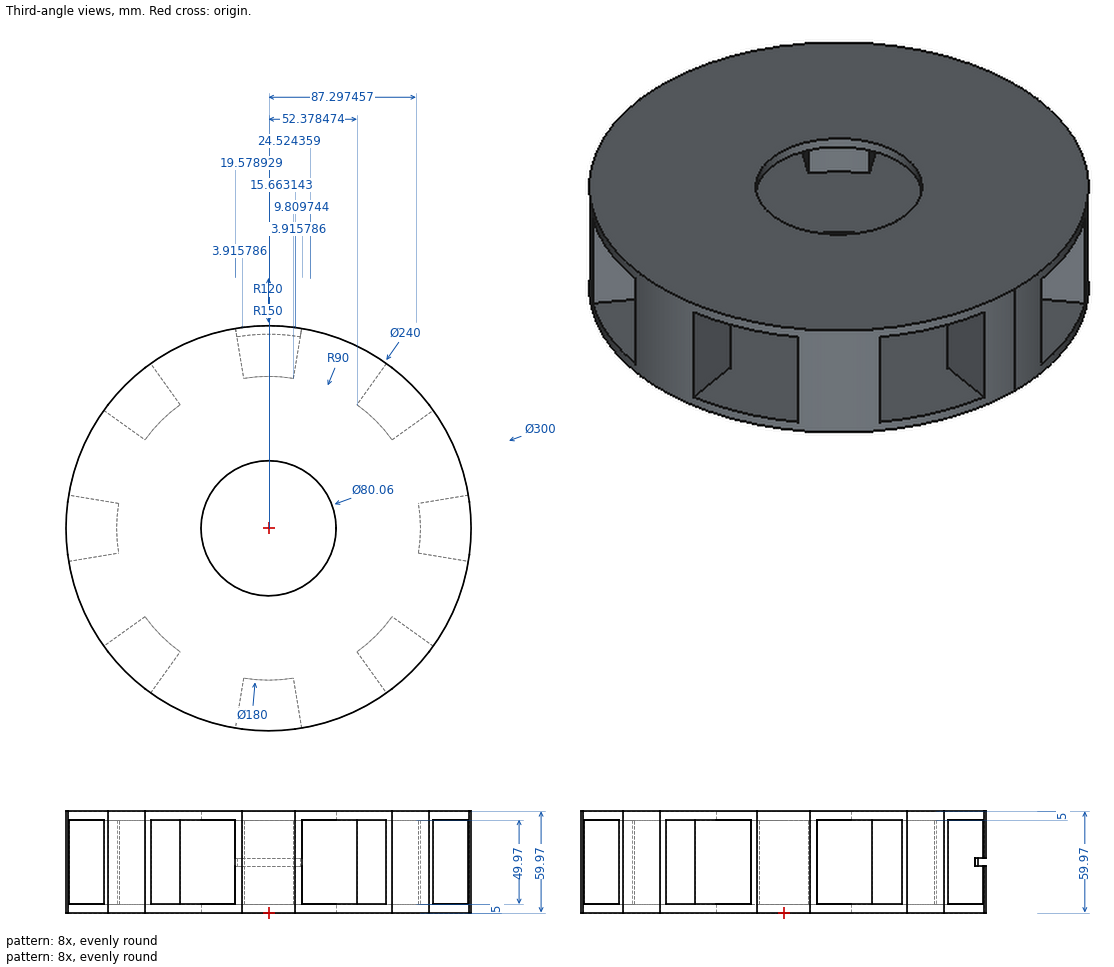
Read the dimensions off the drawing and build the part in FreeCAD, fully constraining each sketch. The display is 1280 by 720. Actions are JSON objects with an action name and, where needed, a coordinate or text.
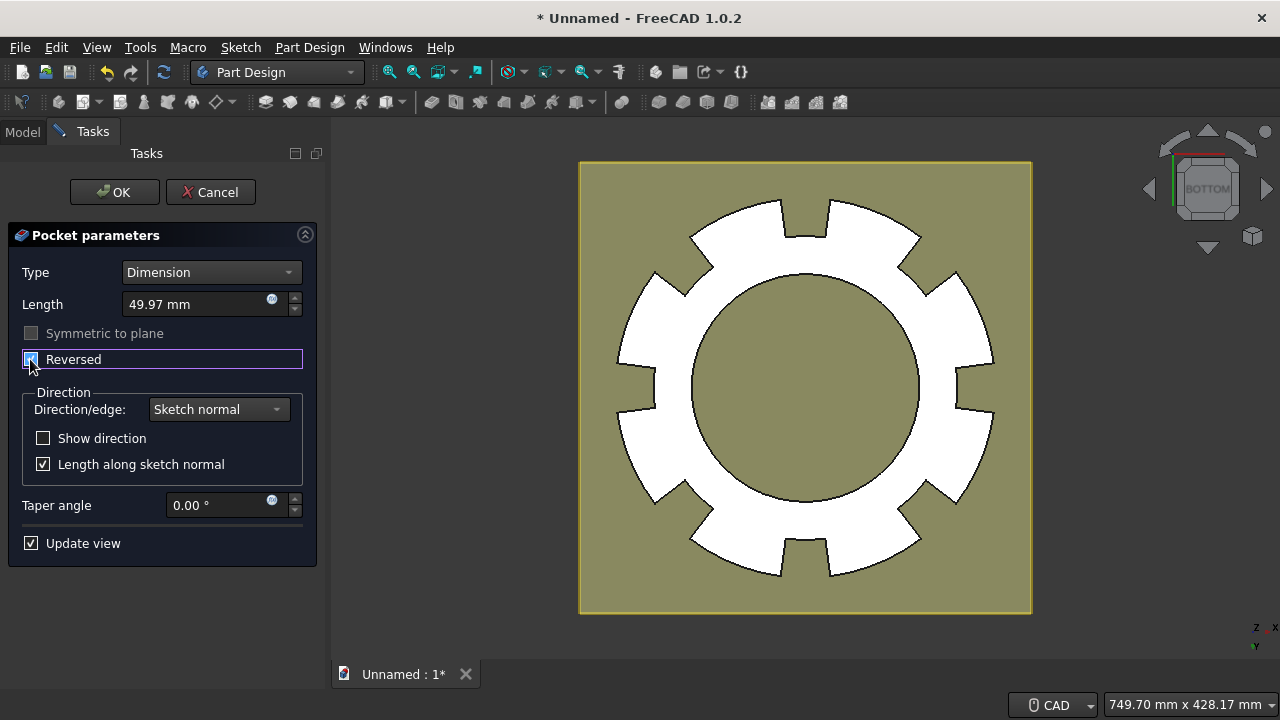
{"action": "left_click", "coordinate": [115, 192]}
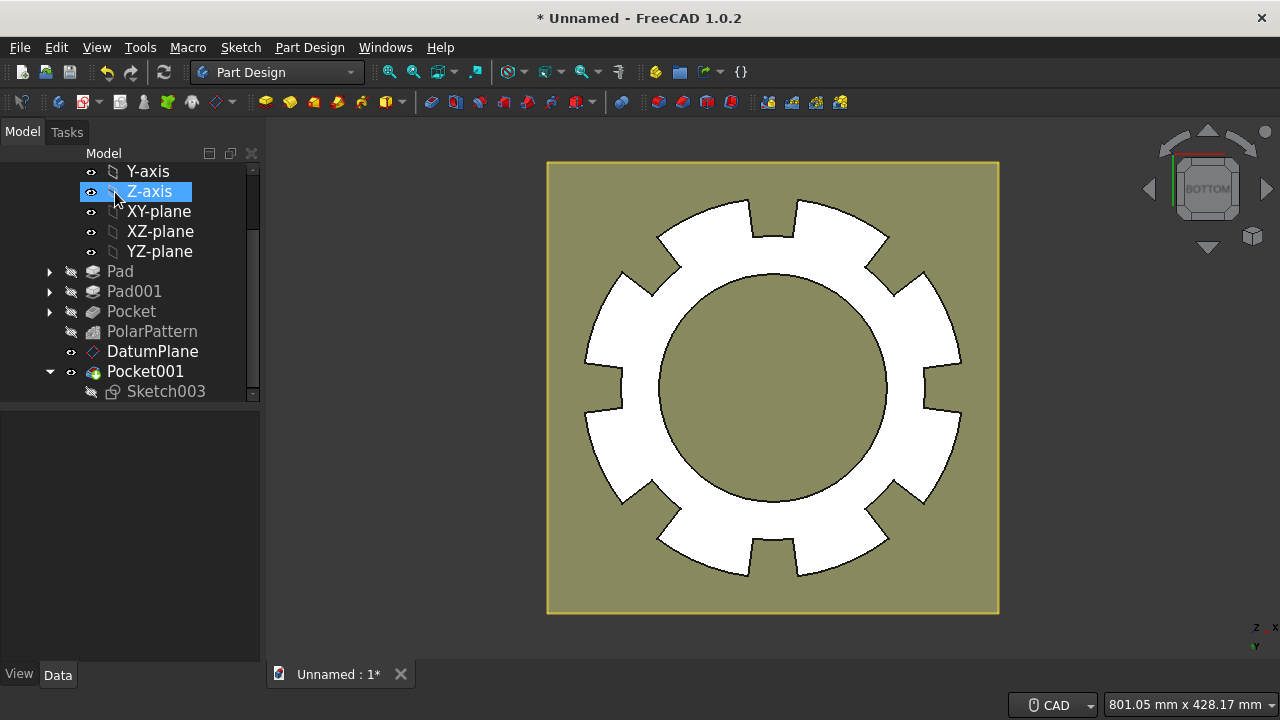
{"action": "left_click", "coordinate": [116, 352]}
{"action": "key", "text": "space"}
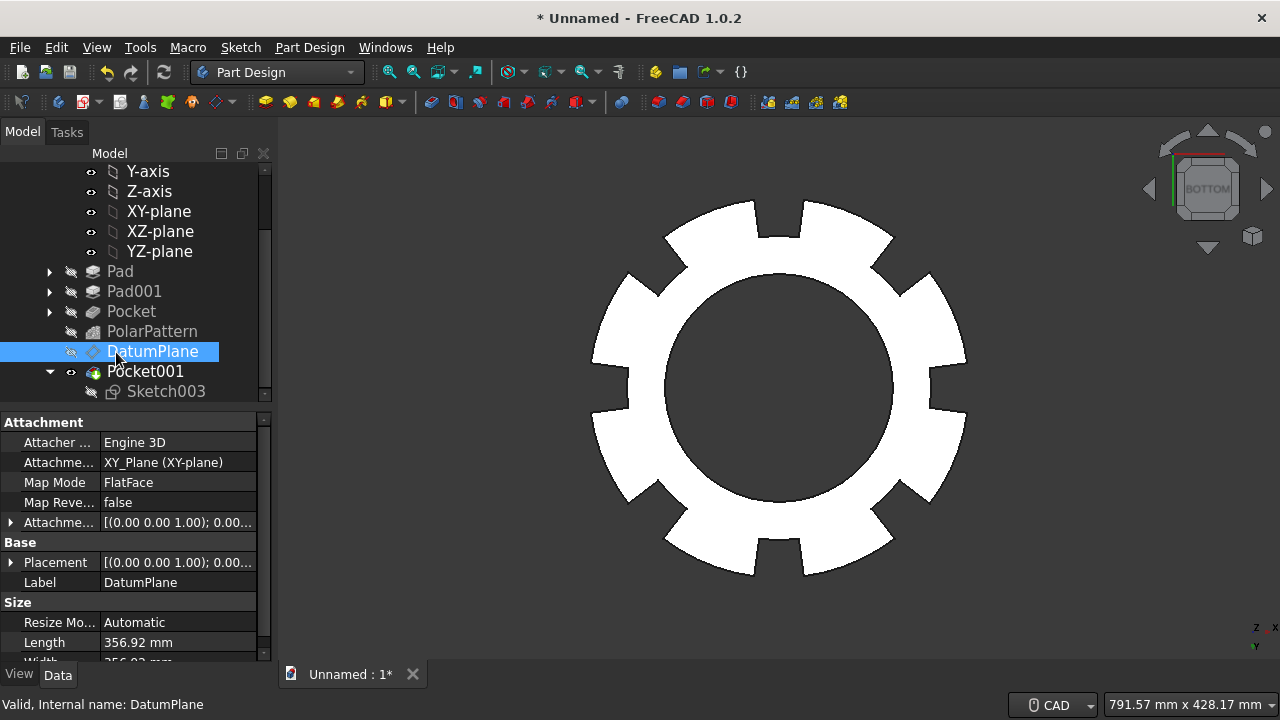
{"action": "left_click", "coordinate": [116, 372]}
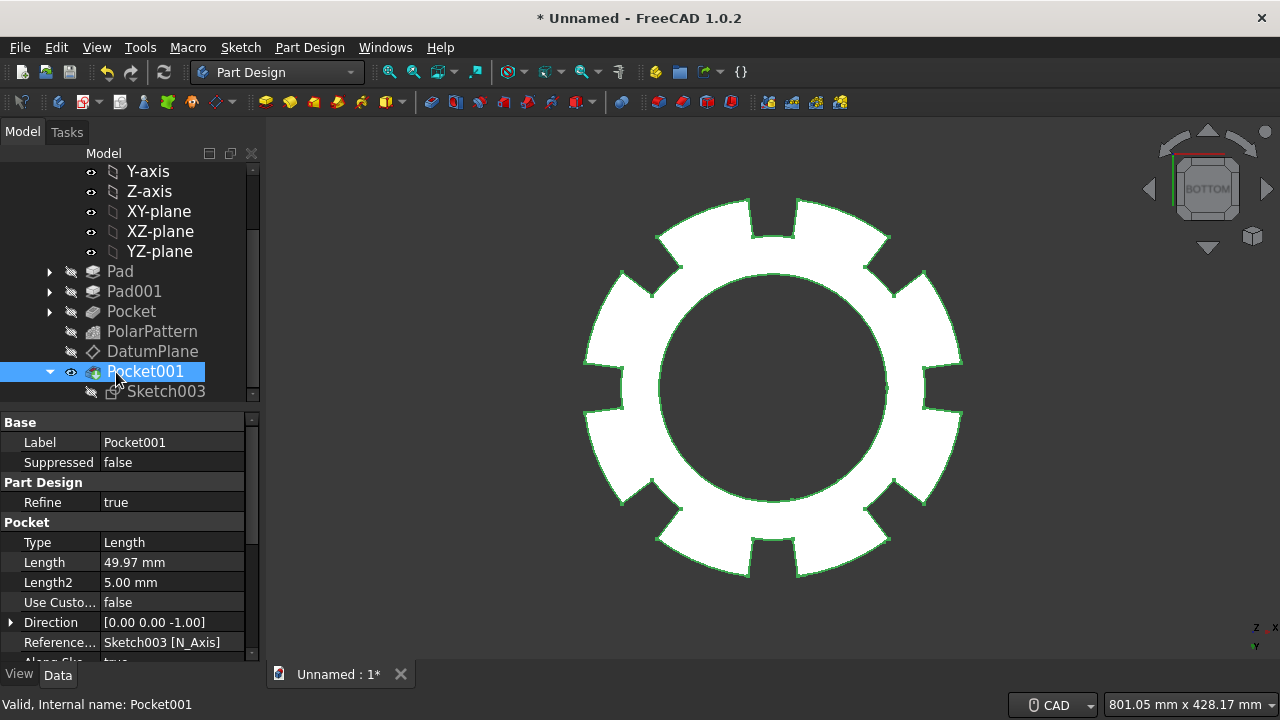
{"action": "left_click", "coordinate": [816, 102]}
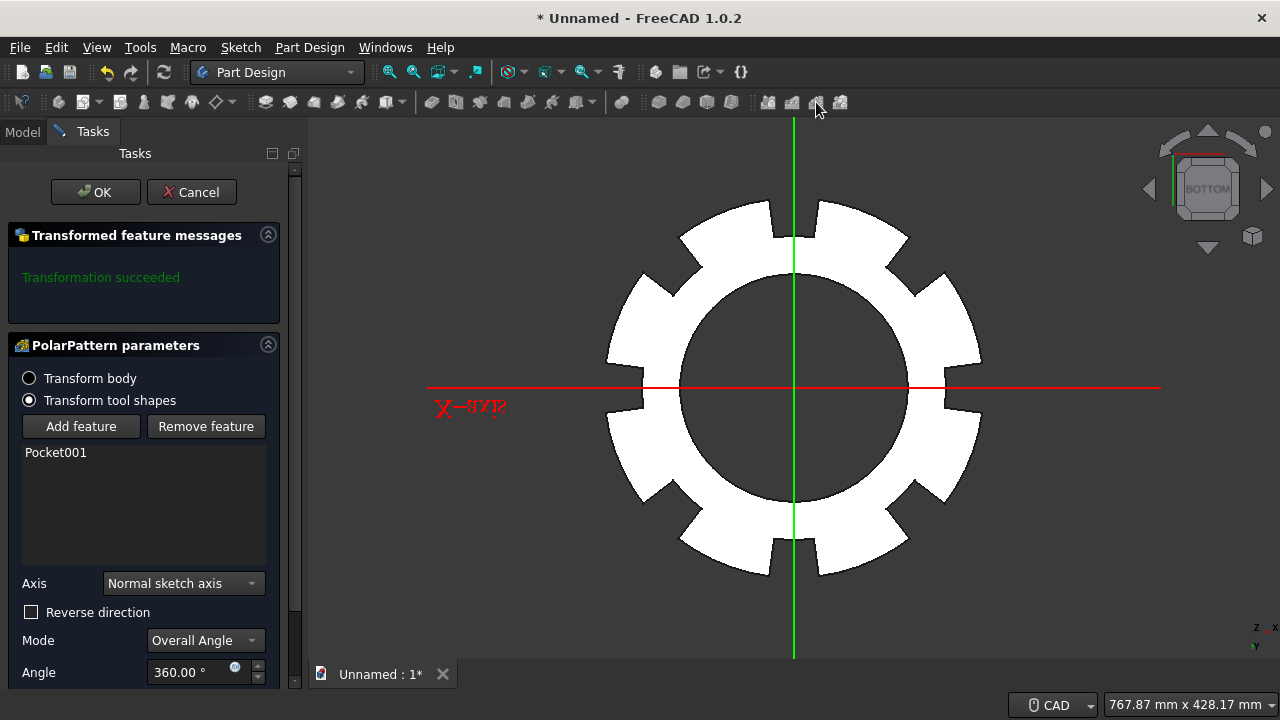
{"action": "left_click", "coordinate": [184, 584]}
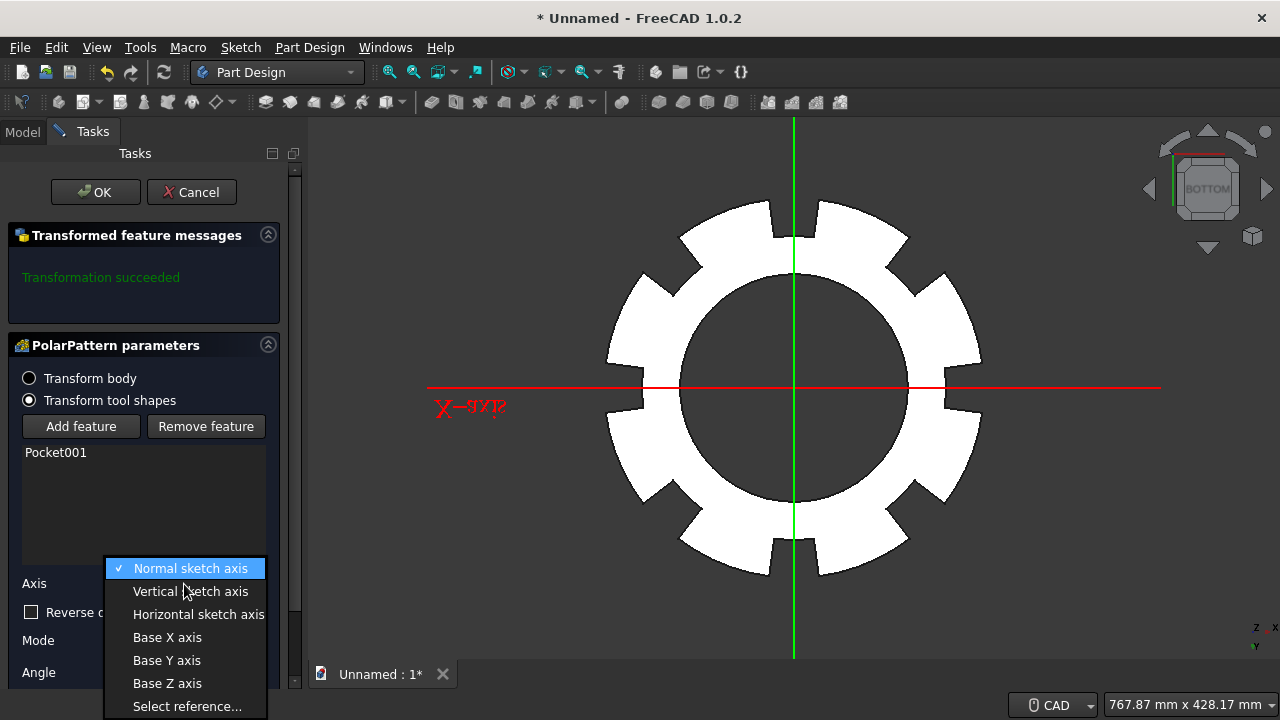
{"action": "left_click", "coordinate": [184, 684]}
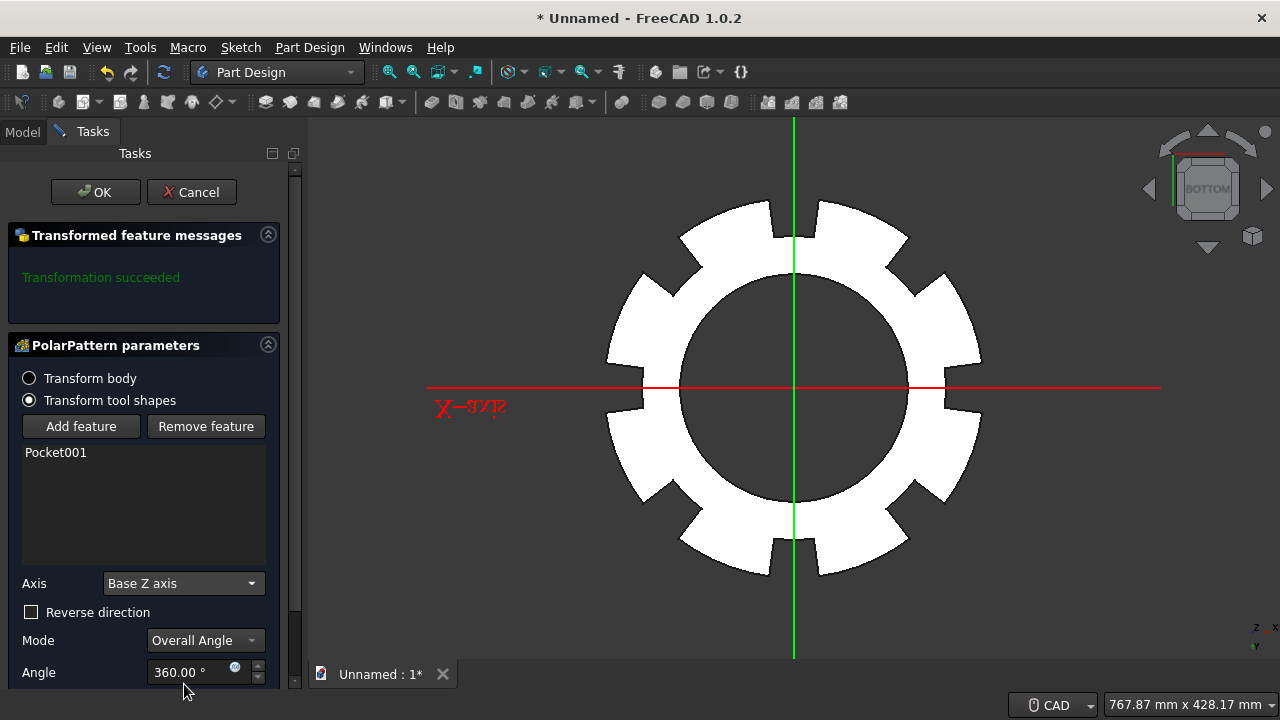
{"action": "scroll", "coordinate": [295, 426], "scroll_direction": "down", "scroll_amount": 2}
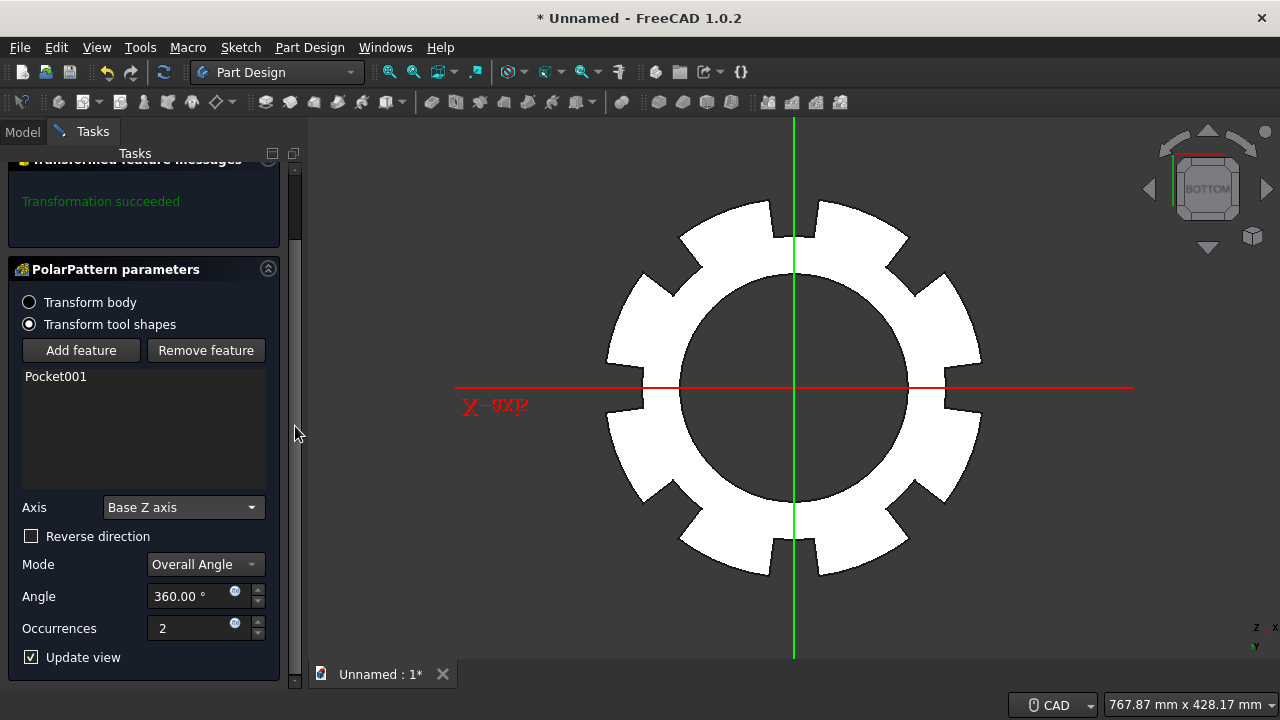
{"action": "triple_click", "coordinate": [198, 628]}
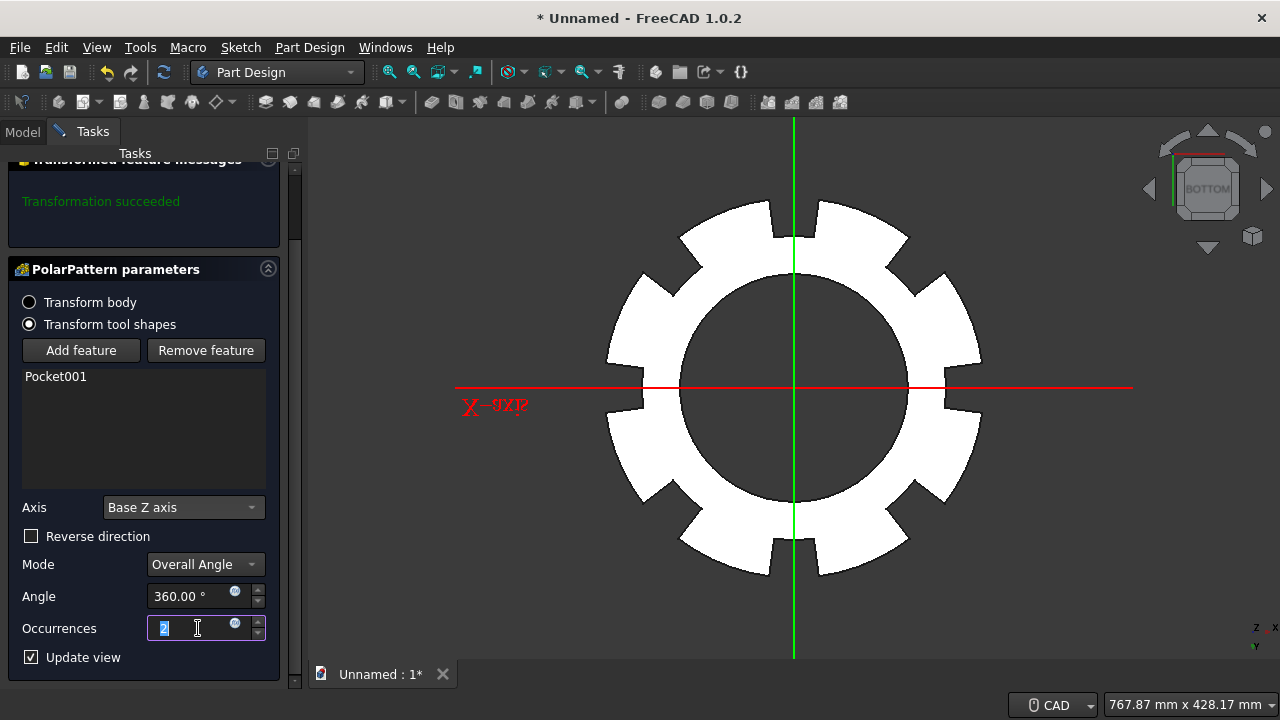
{"action": "type", "text": "8"}
{"action": "key", "text": "Tab"}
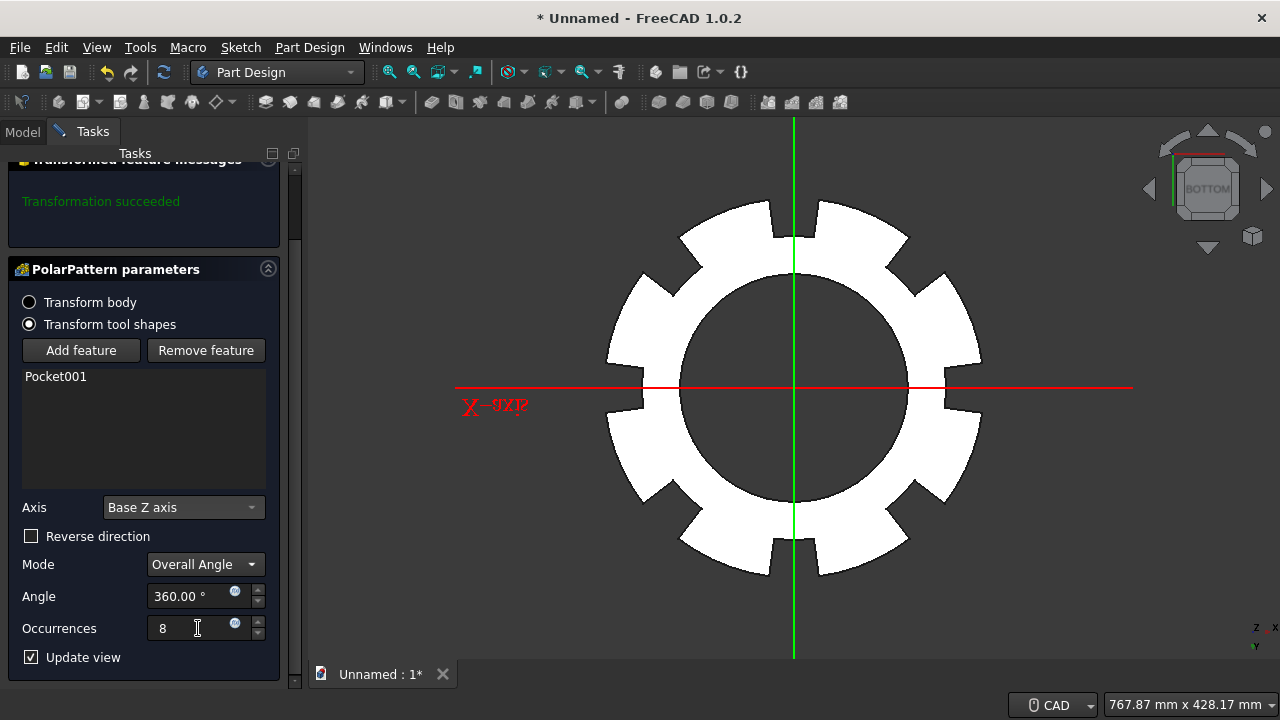
{"action": "scroll", "coordinate": [295, 426], "scroll_direction": "up", "scroll_amount": 3}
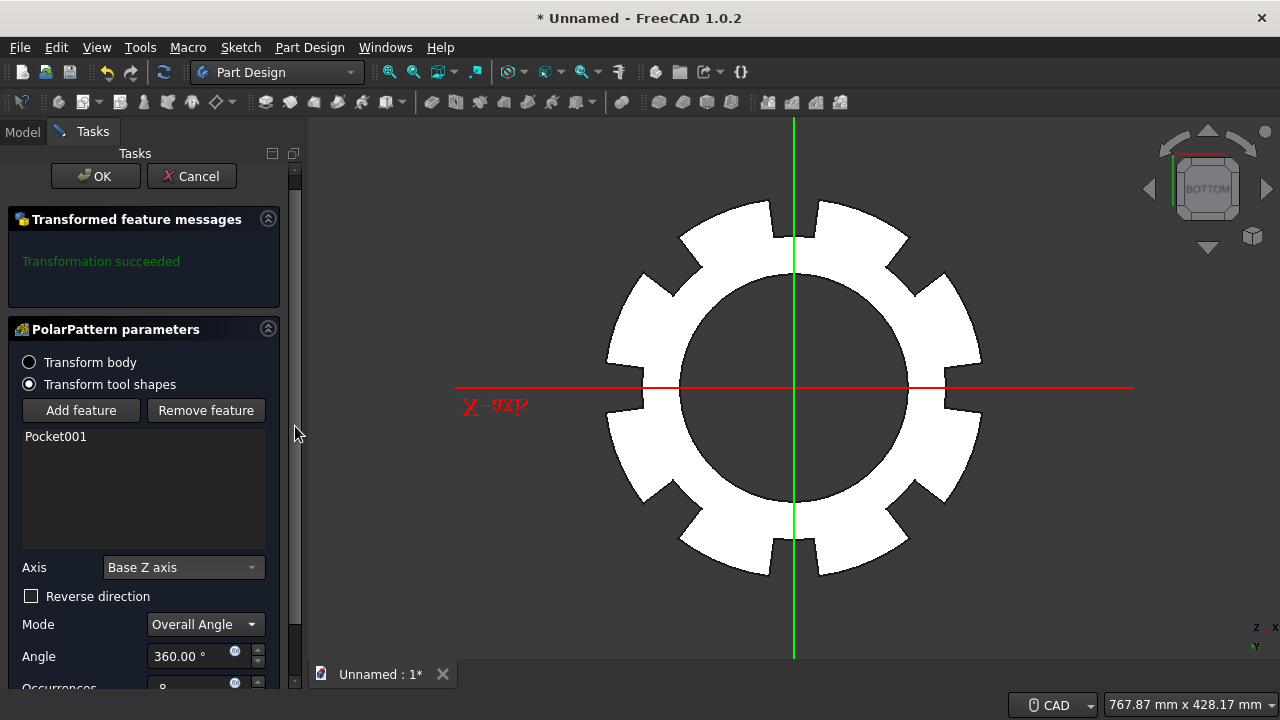
{"action": "left_click", "coordinate": [96, 192]}